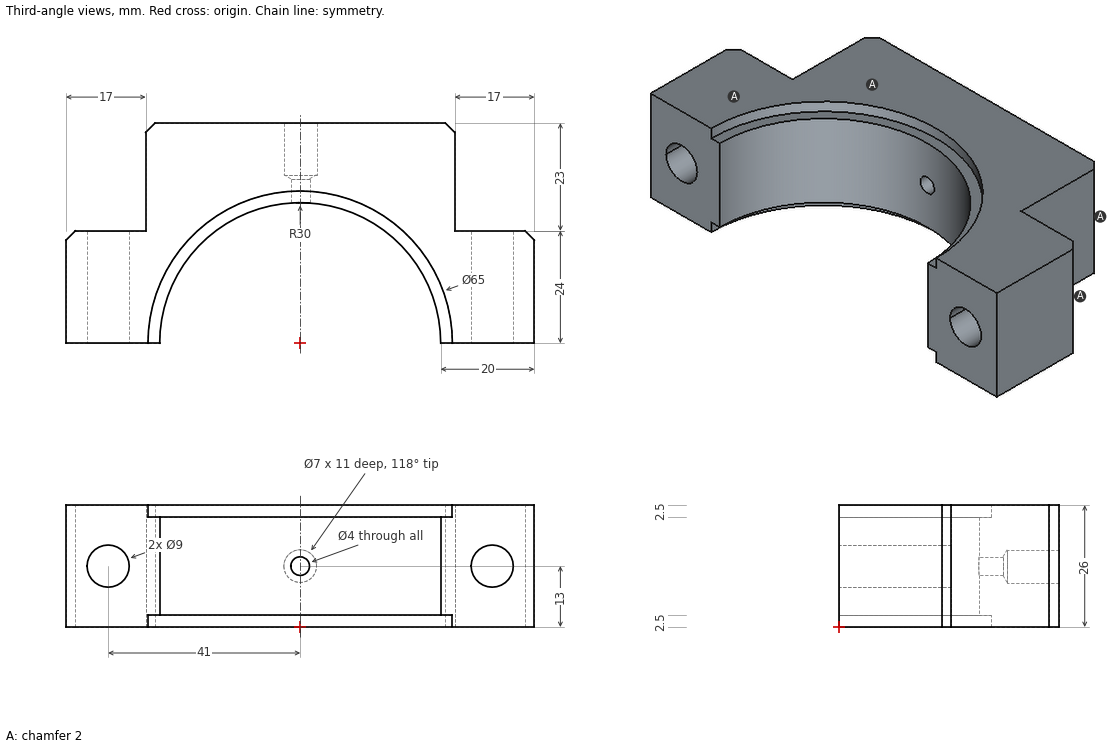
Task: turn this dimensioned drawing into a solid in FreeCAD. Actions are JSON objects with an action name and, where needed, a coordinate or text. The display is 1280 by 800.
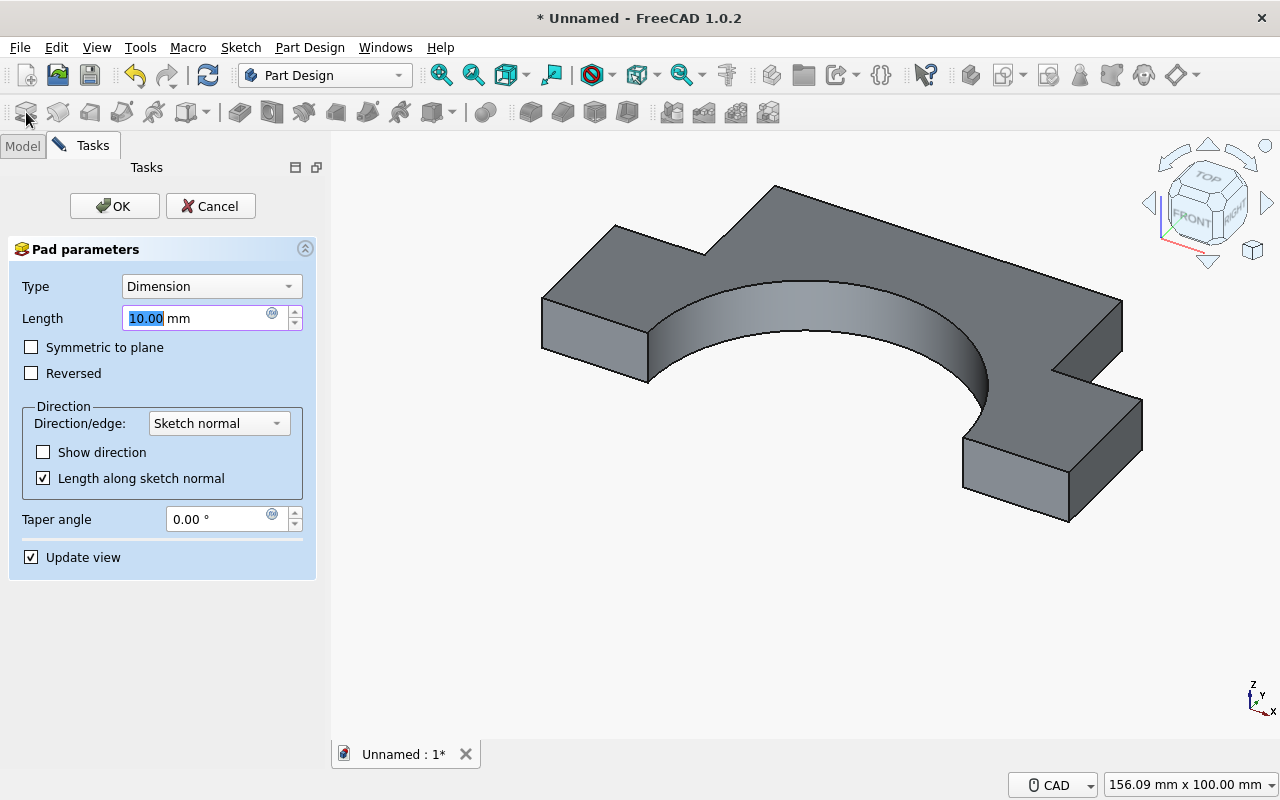
{"action": "type", "text": "26"}
{"action": "key", "text": "Tab"}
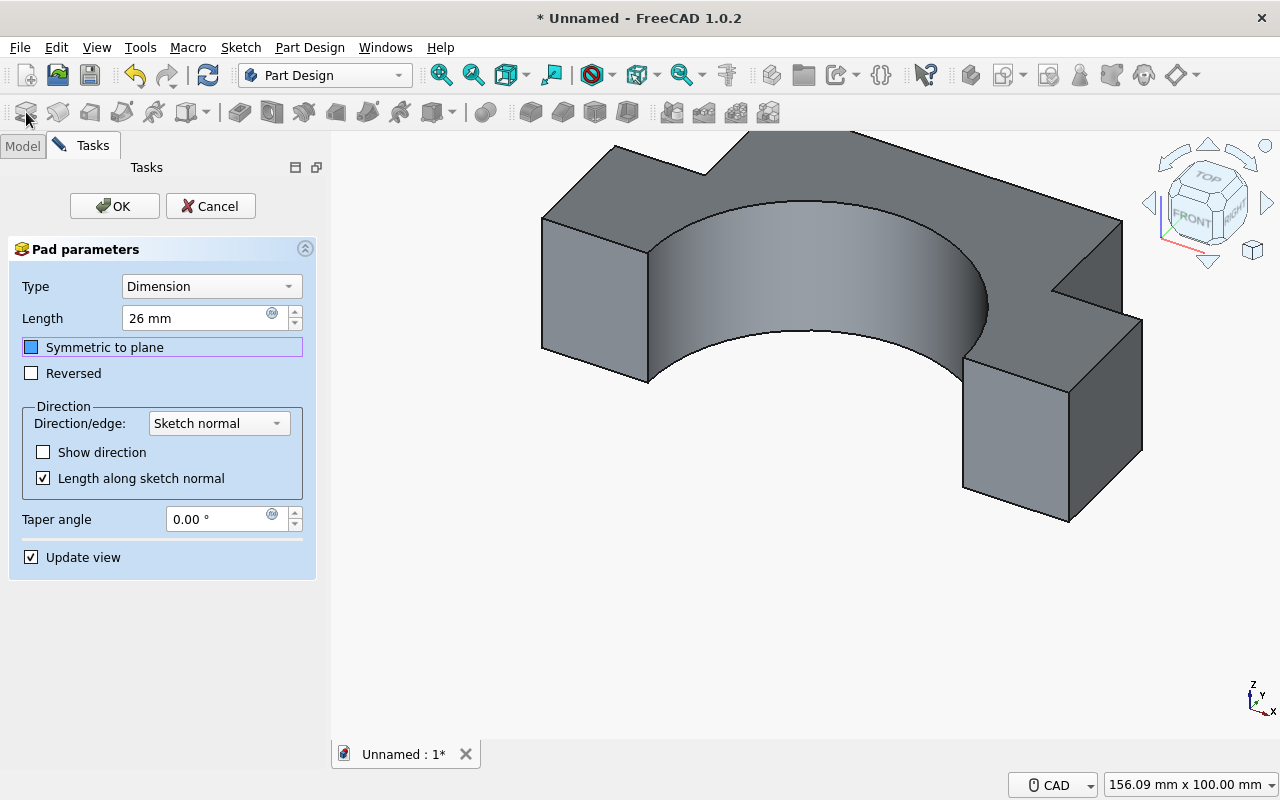
{"action": "left_click", "coordinate": [115, 206]}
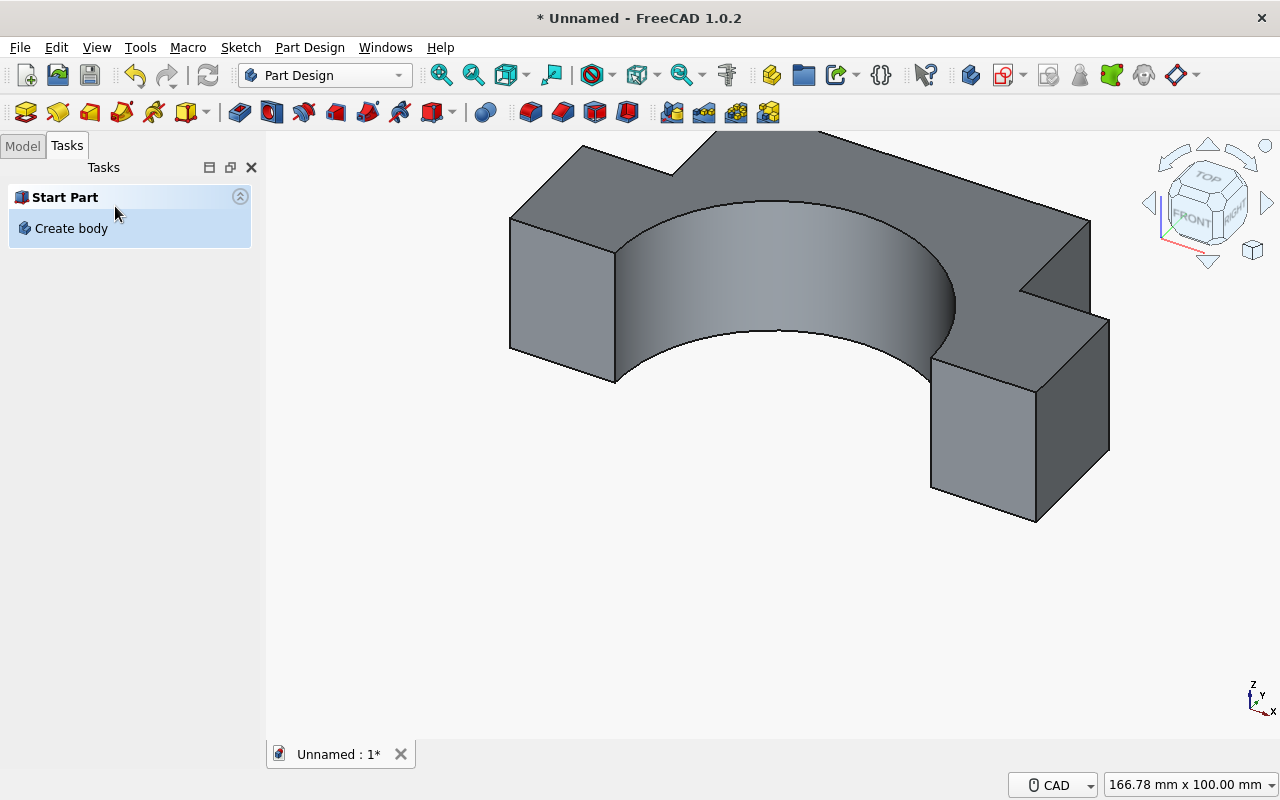
{"action": "left_click", "coordinate": [442, 76]}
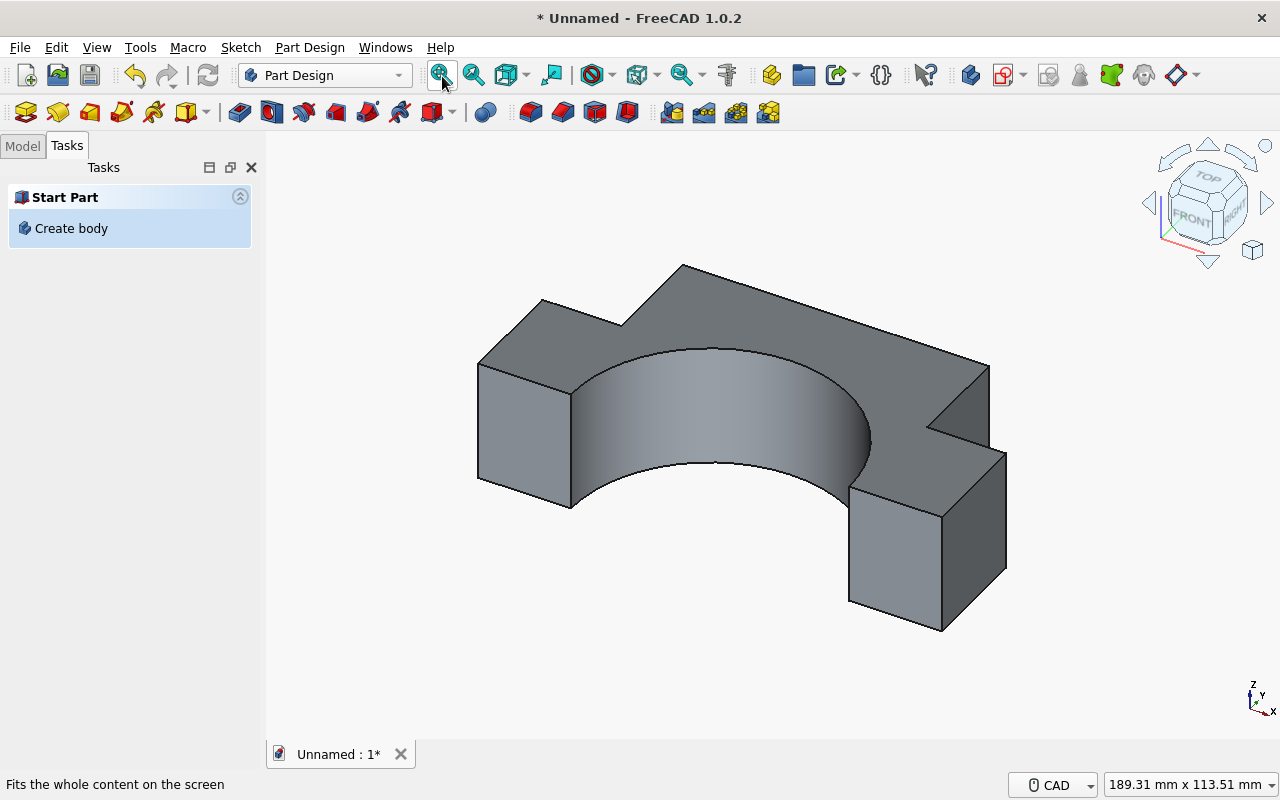
{"action": "key", "text": "0"}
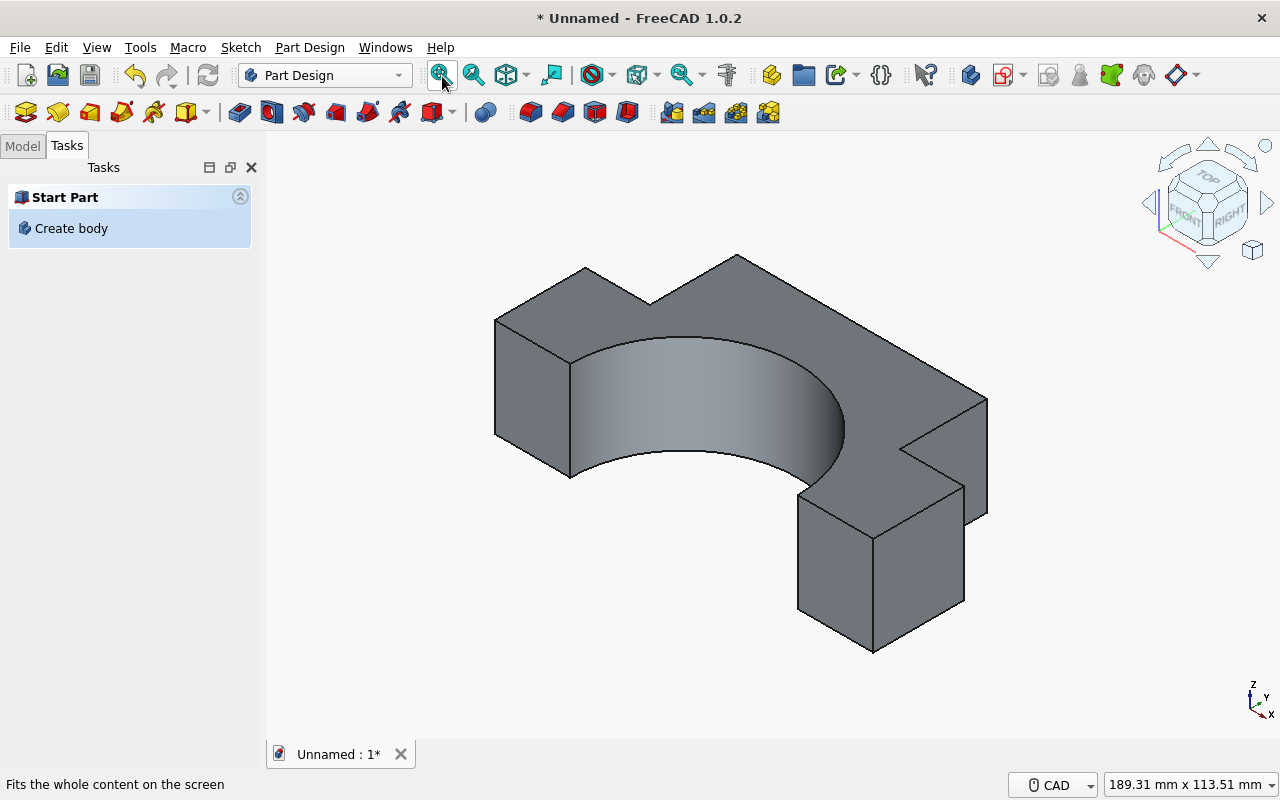
{"action": "key", "text": "2"}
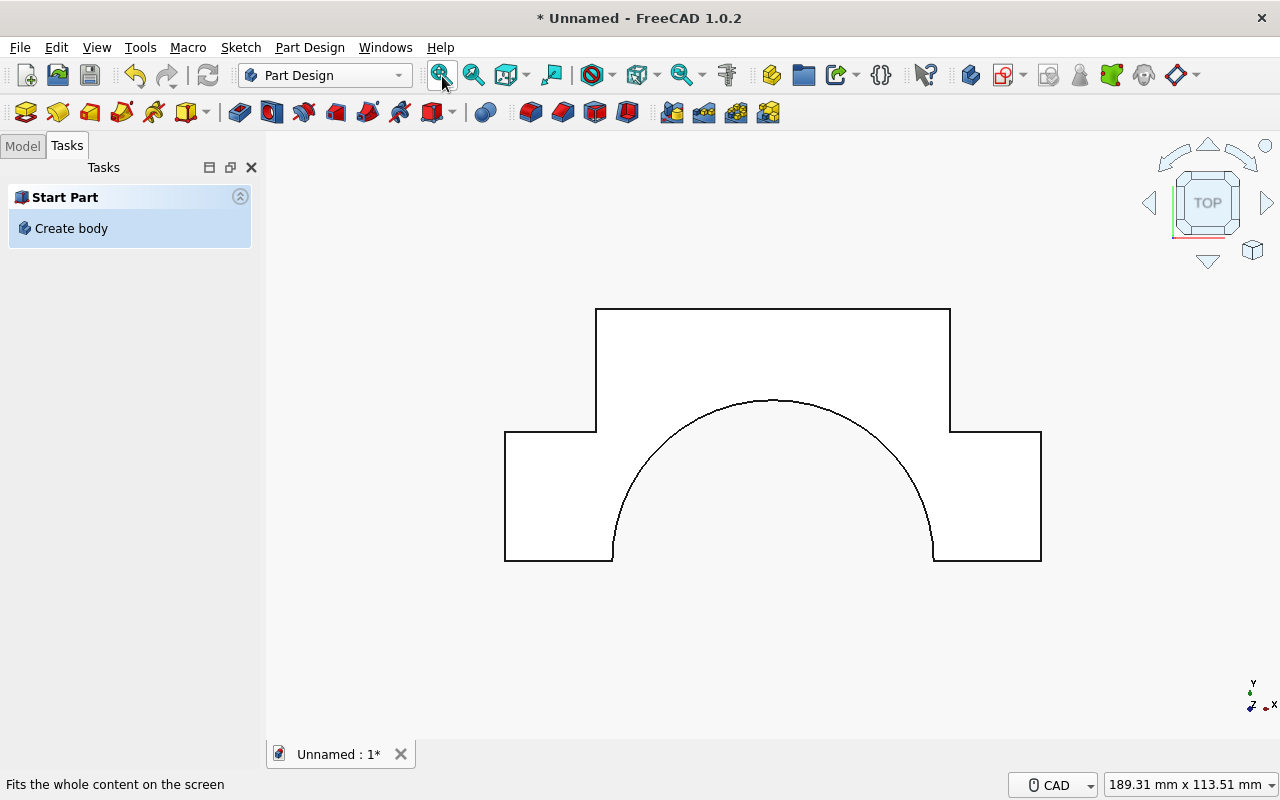
{"action": "key", "text": "1"}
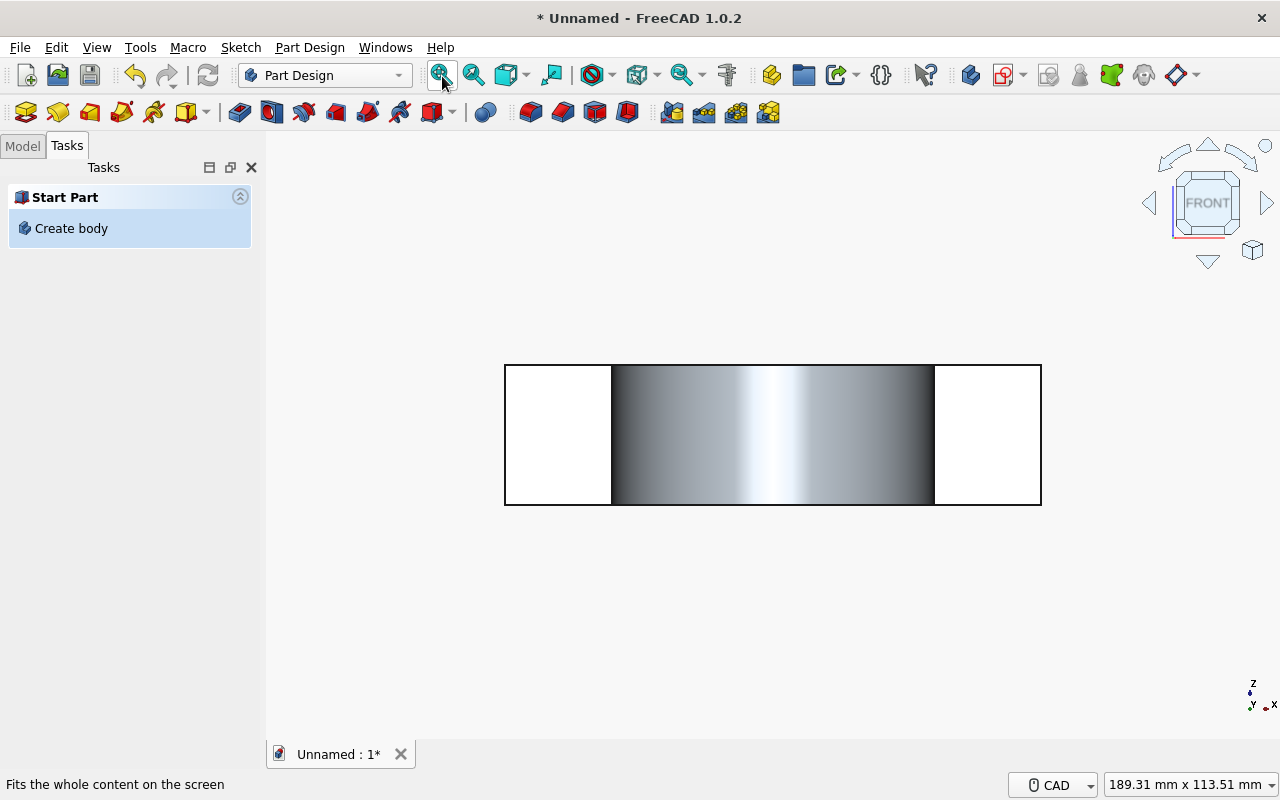
{"action": "key", "text": "3"}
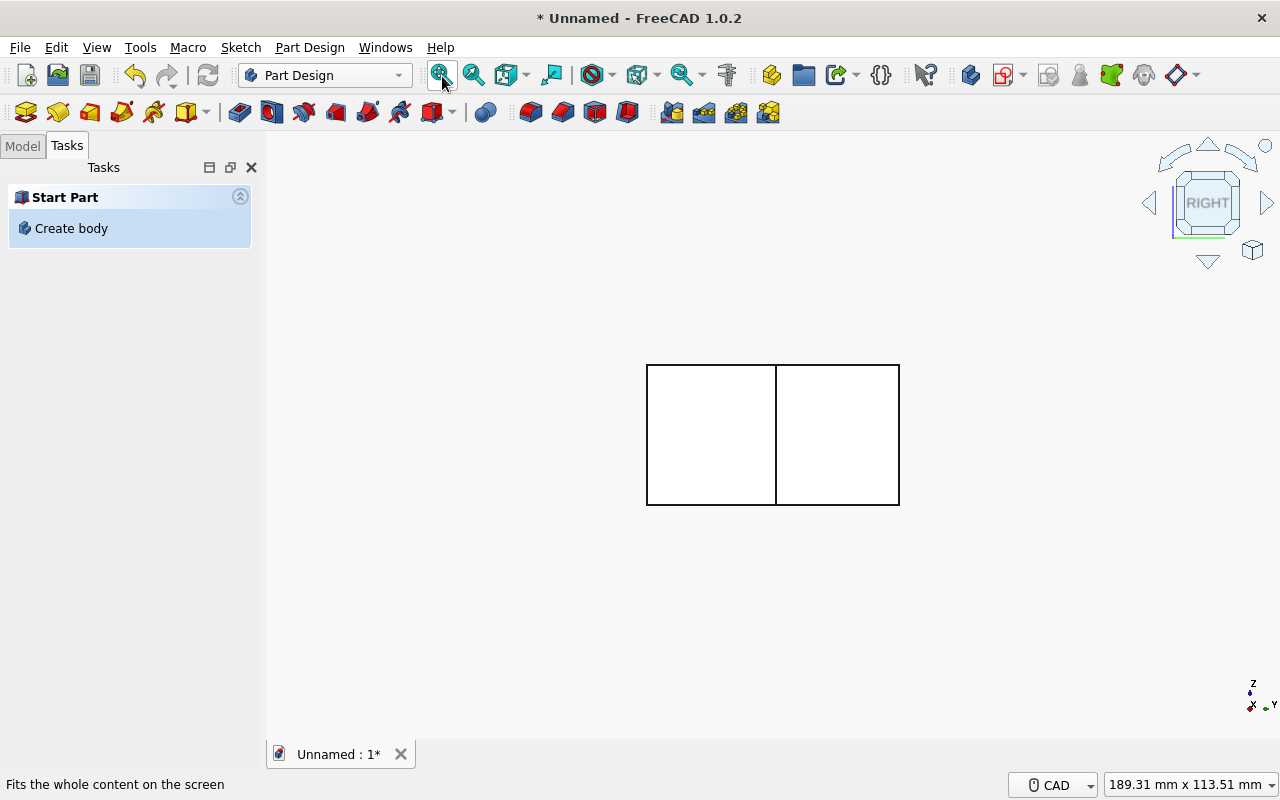
{"action": "key", "text": "v f"}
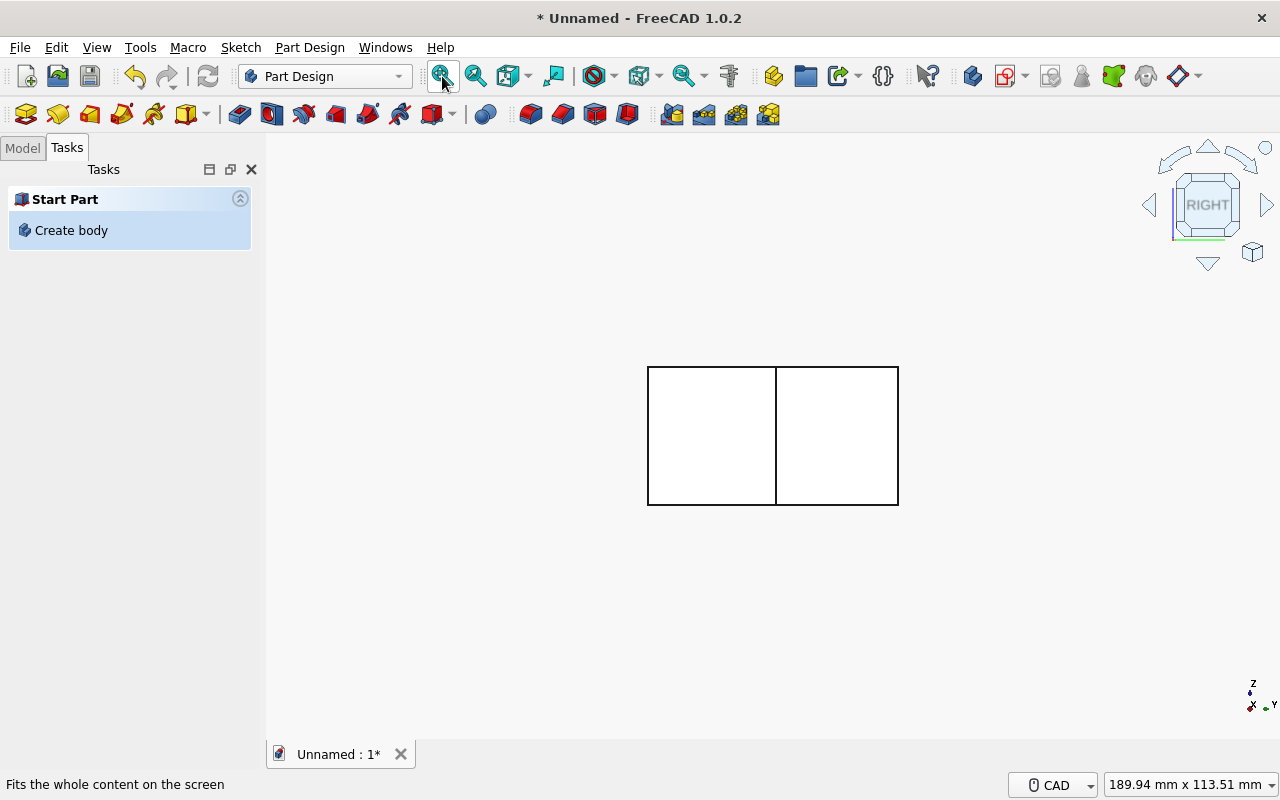
{"action": "left_click", "coordinate": [898, 435]}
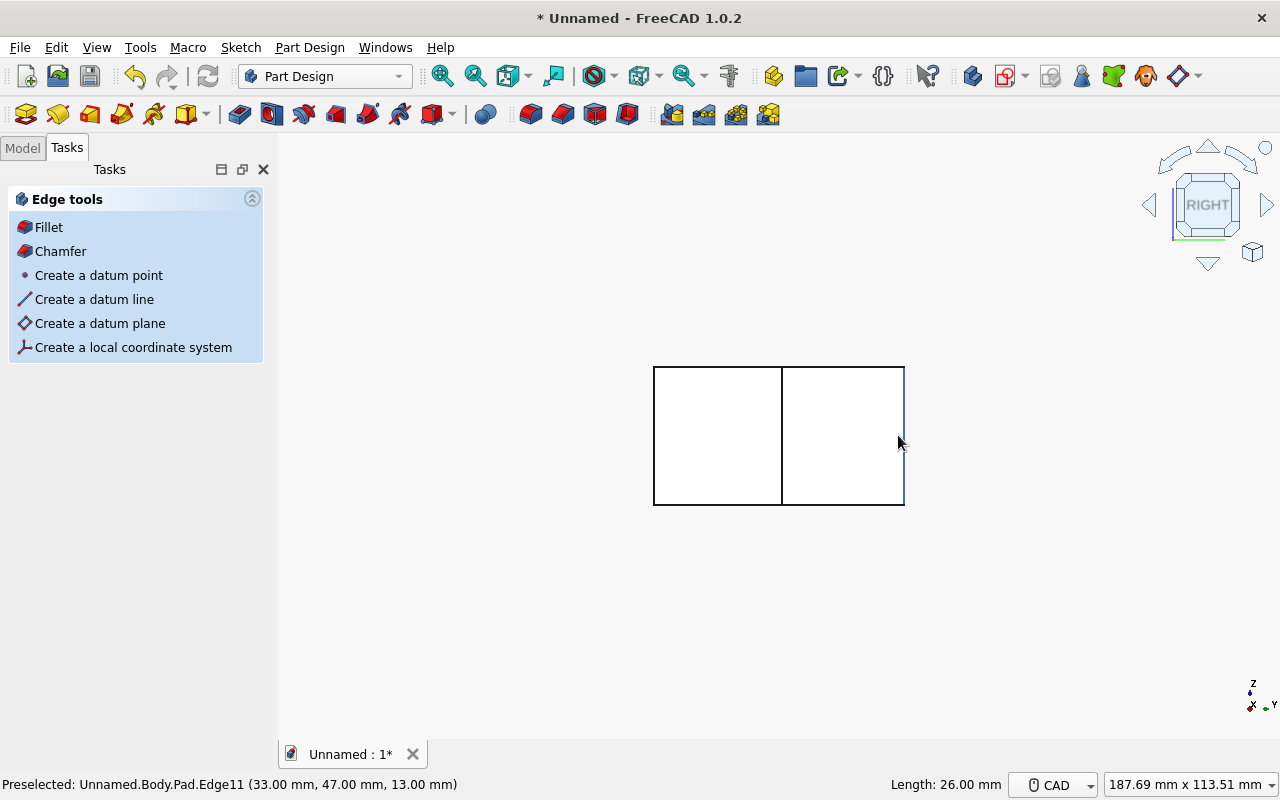
{"action": "left_click", "coordinate": [782, 435], "text": "ctrl"}